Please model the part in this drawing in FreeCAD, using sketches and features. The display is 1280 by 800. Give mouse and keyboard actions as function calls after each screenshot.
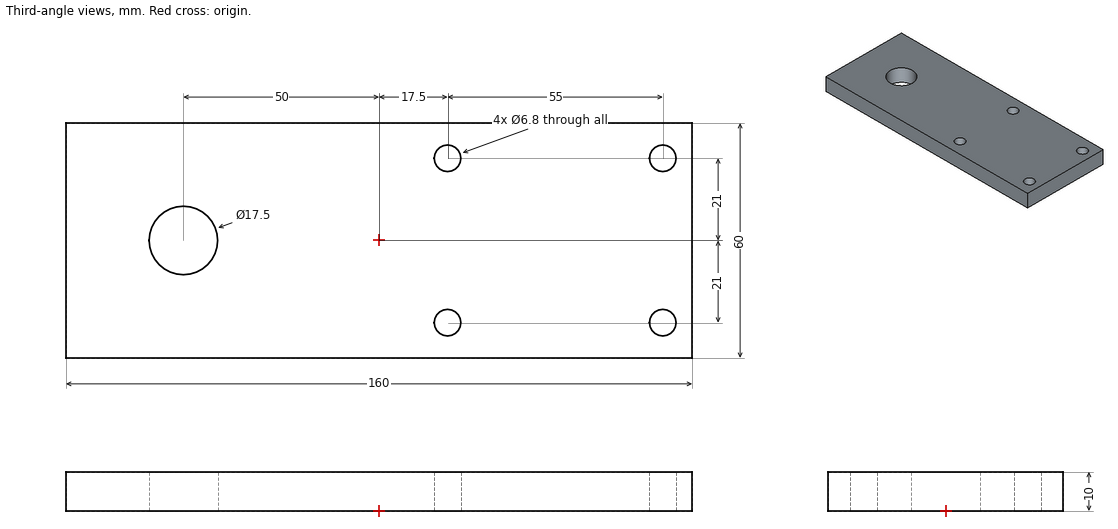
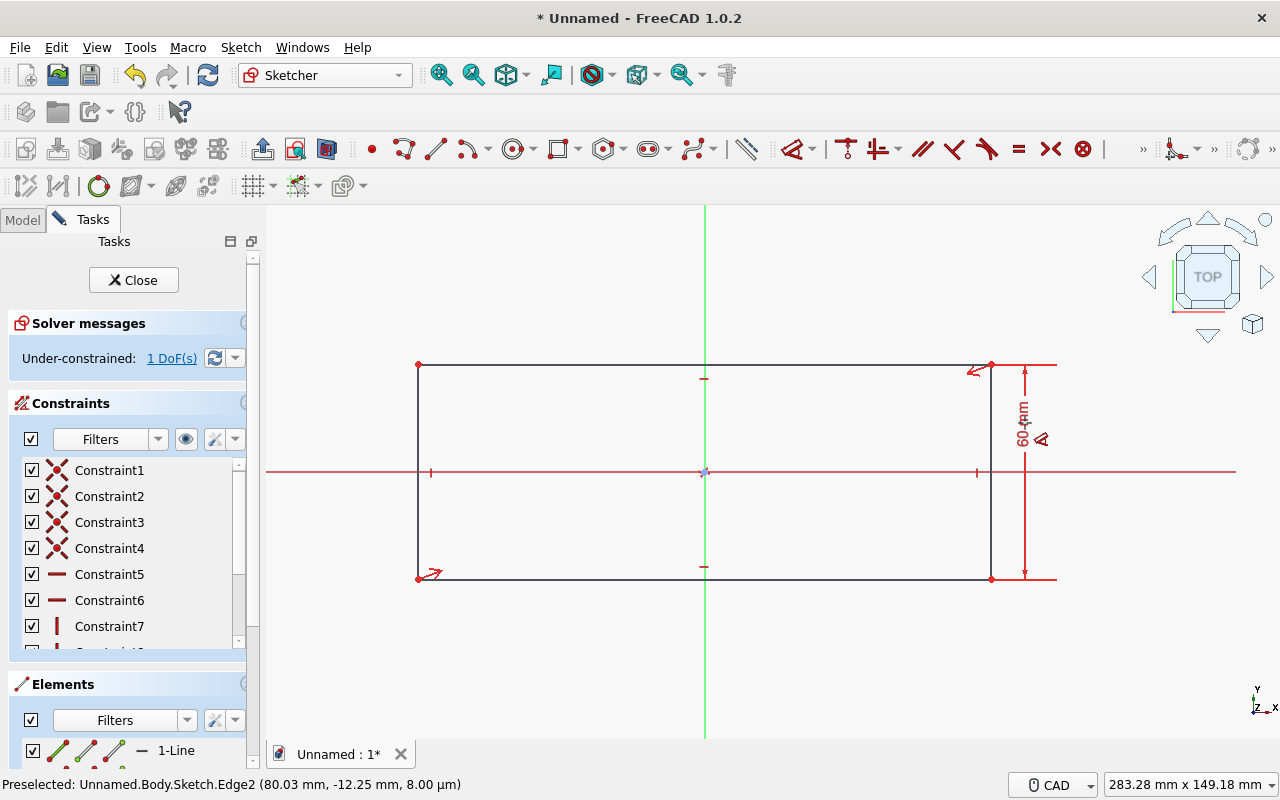
click(590, 580)
click(573, 614)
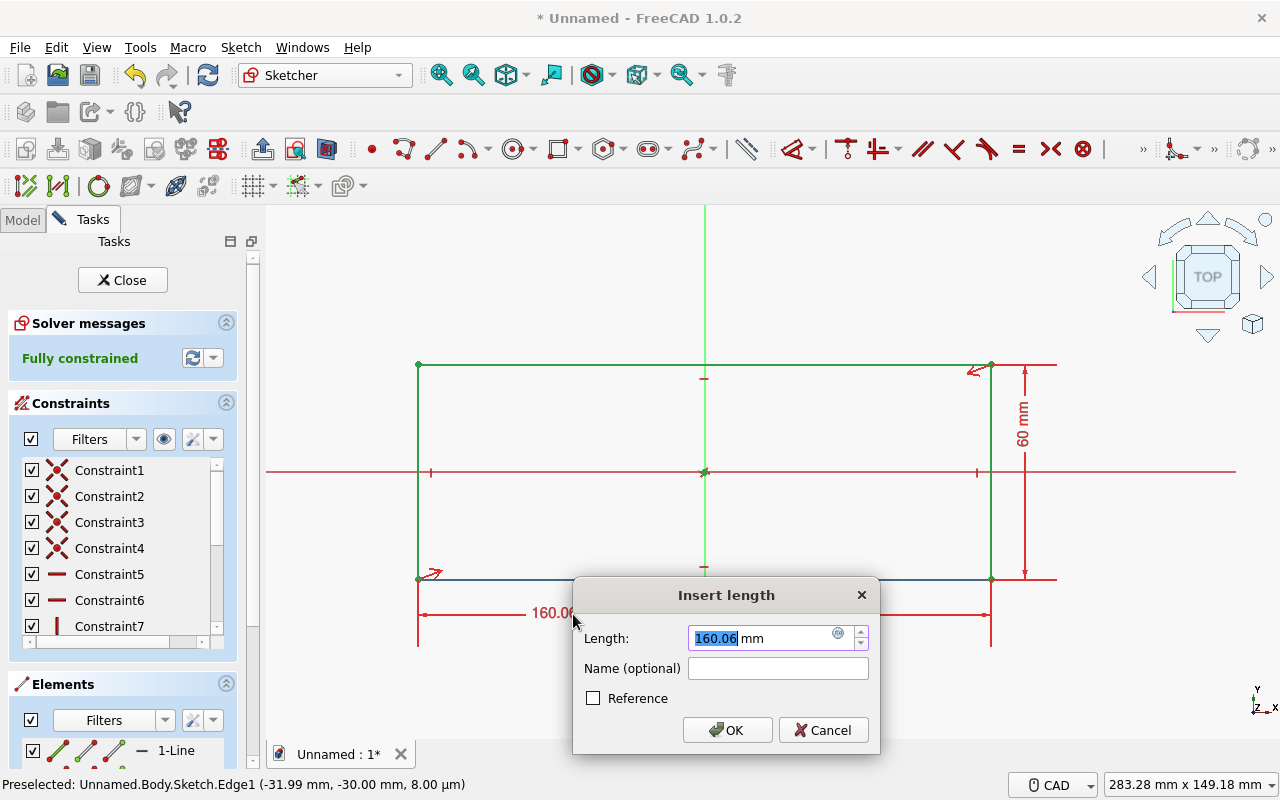
text(160)
key(Return)
key(Escape)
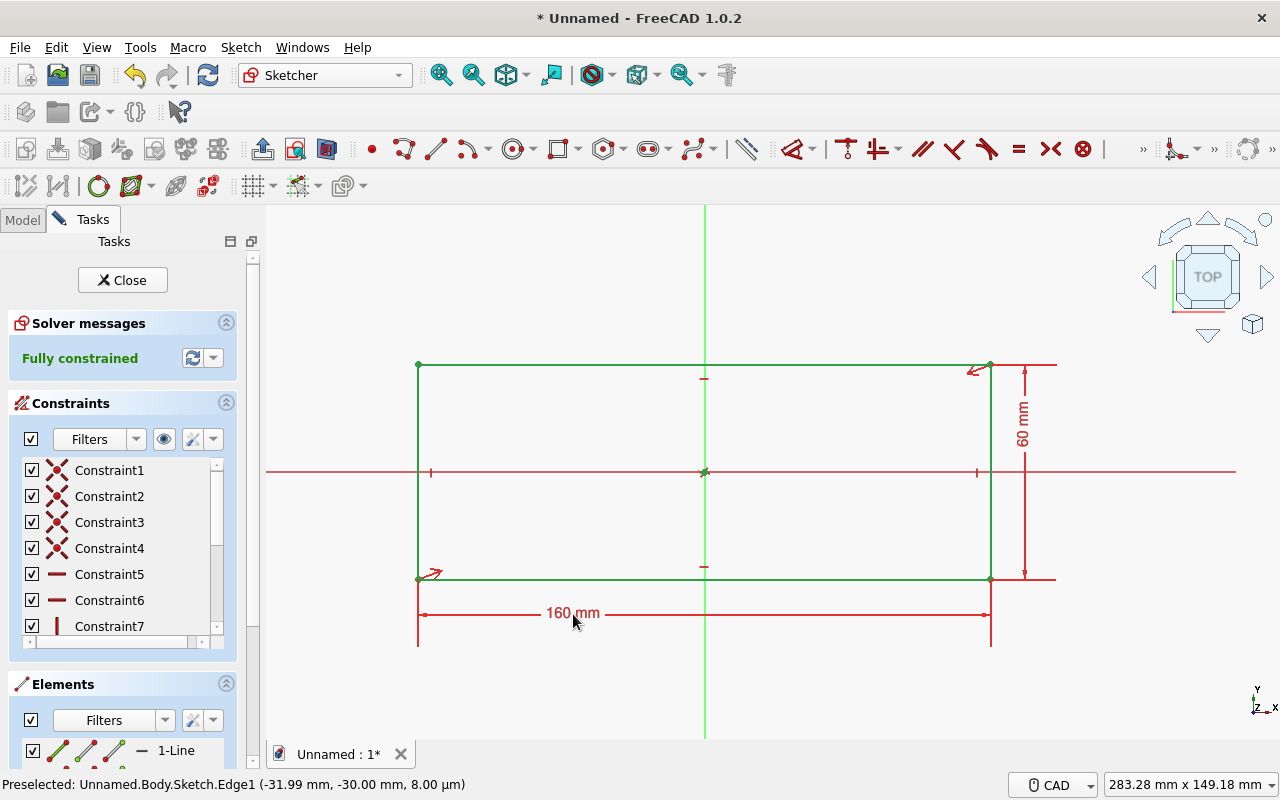
click(123, 280)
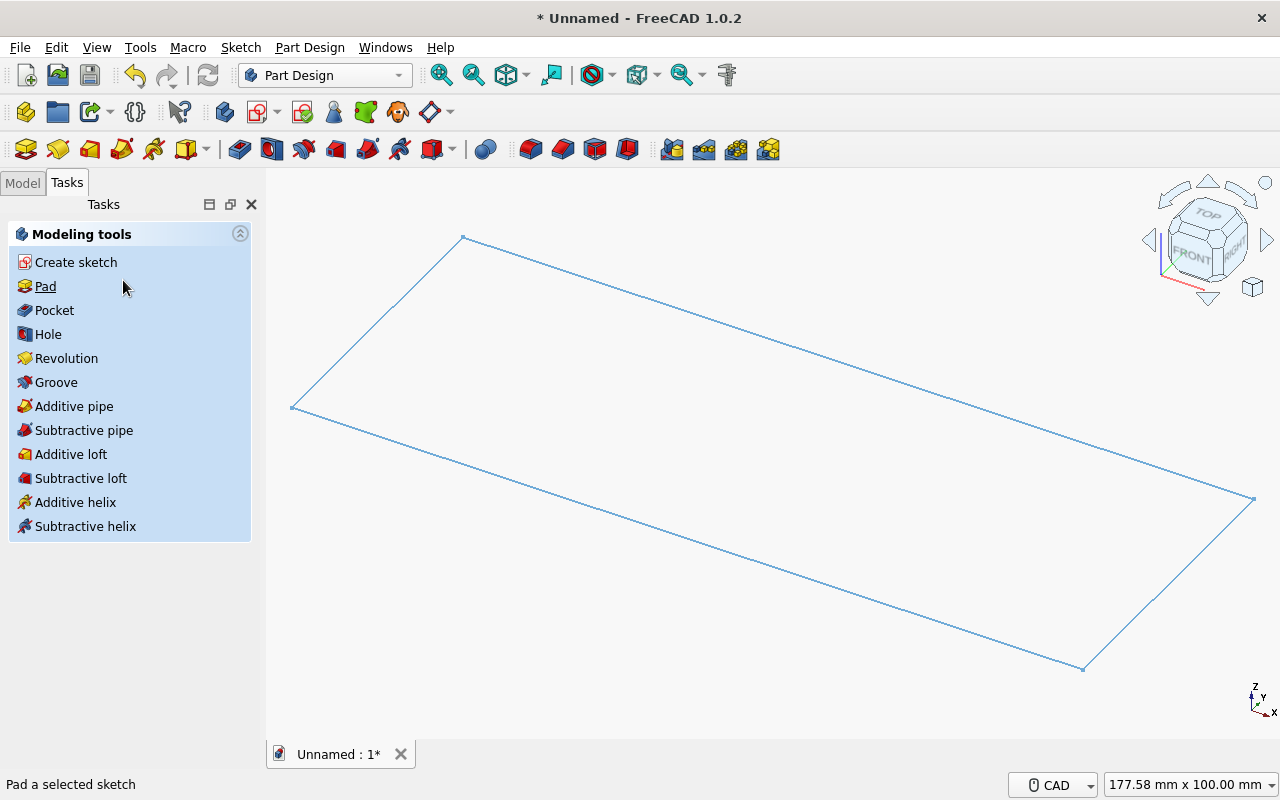
click(26, 150)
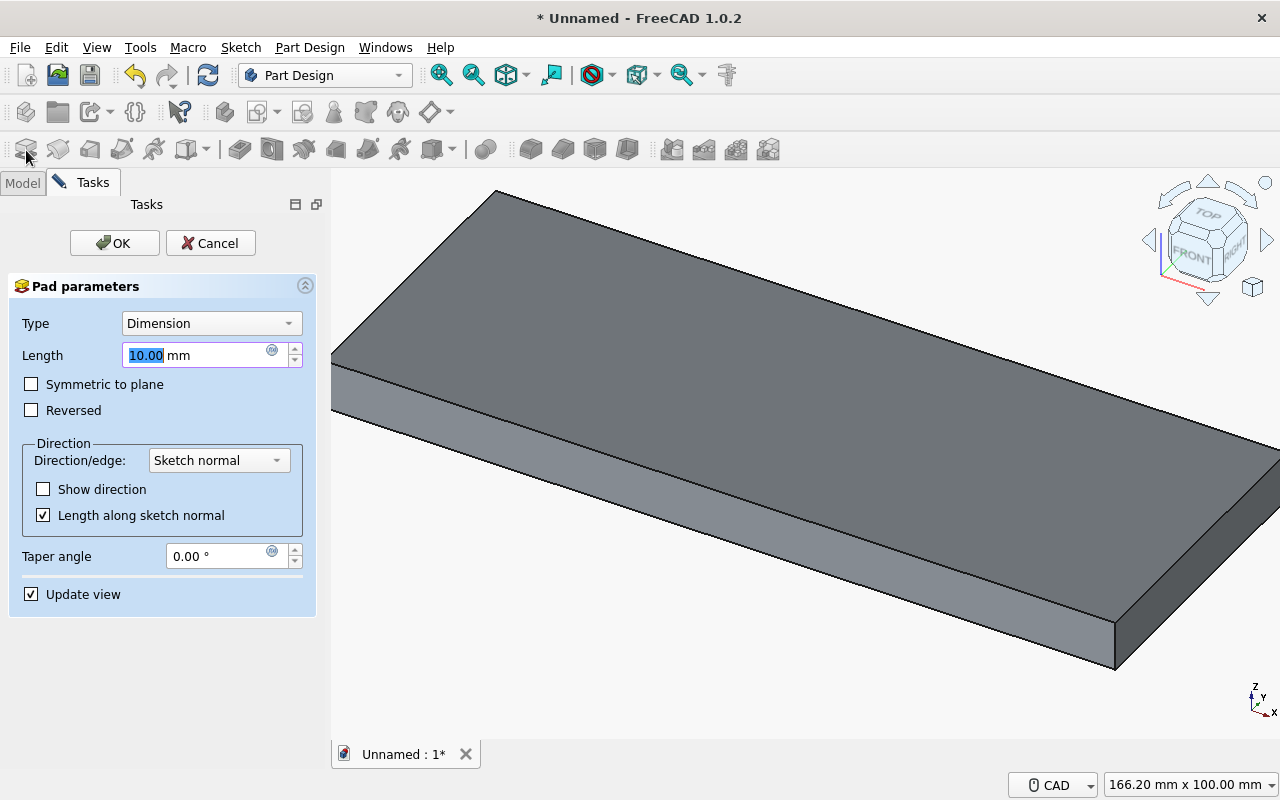
text(10)
key(Tab)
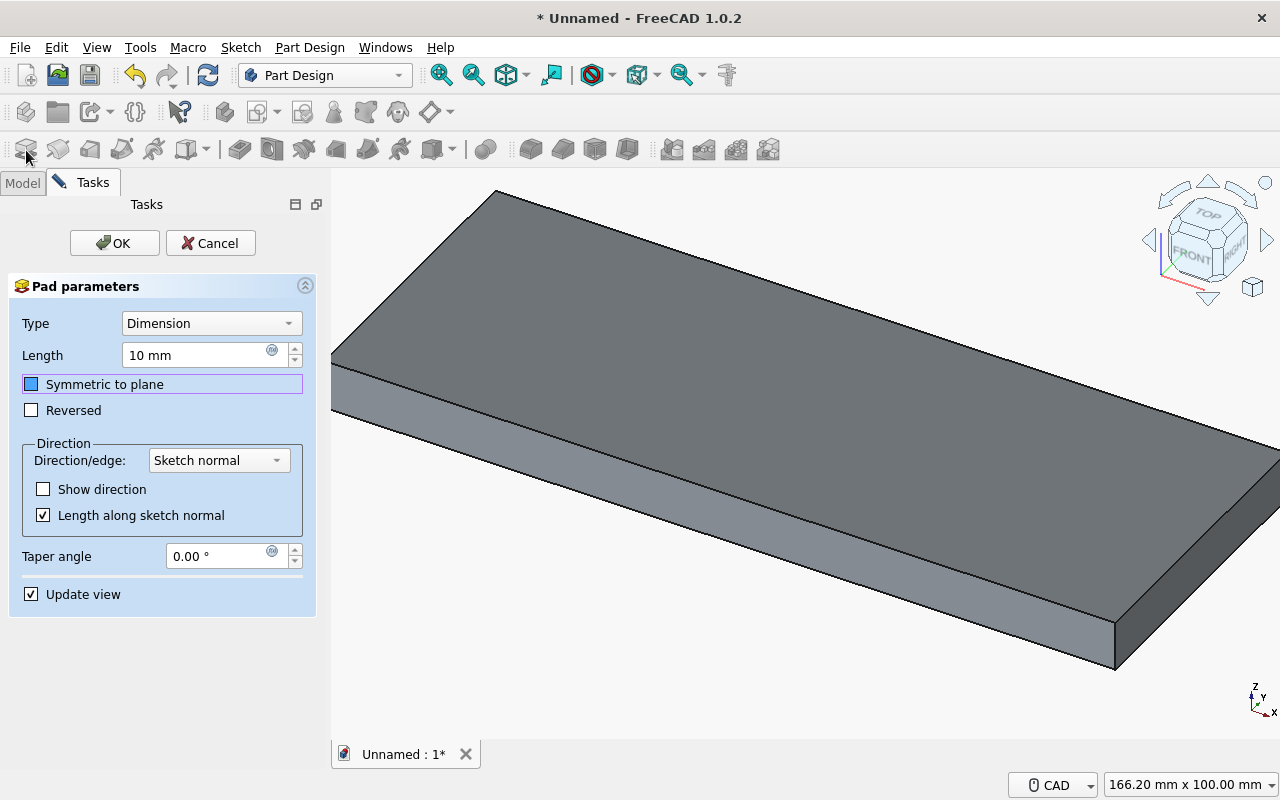
click(115, 243)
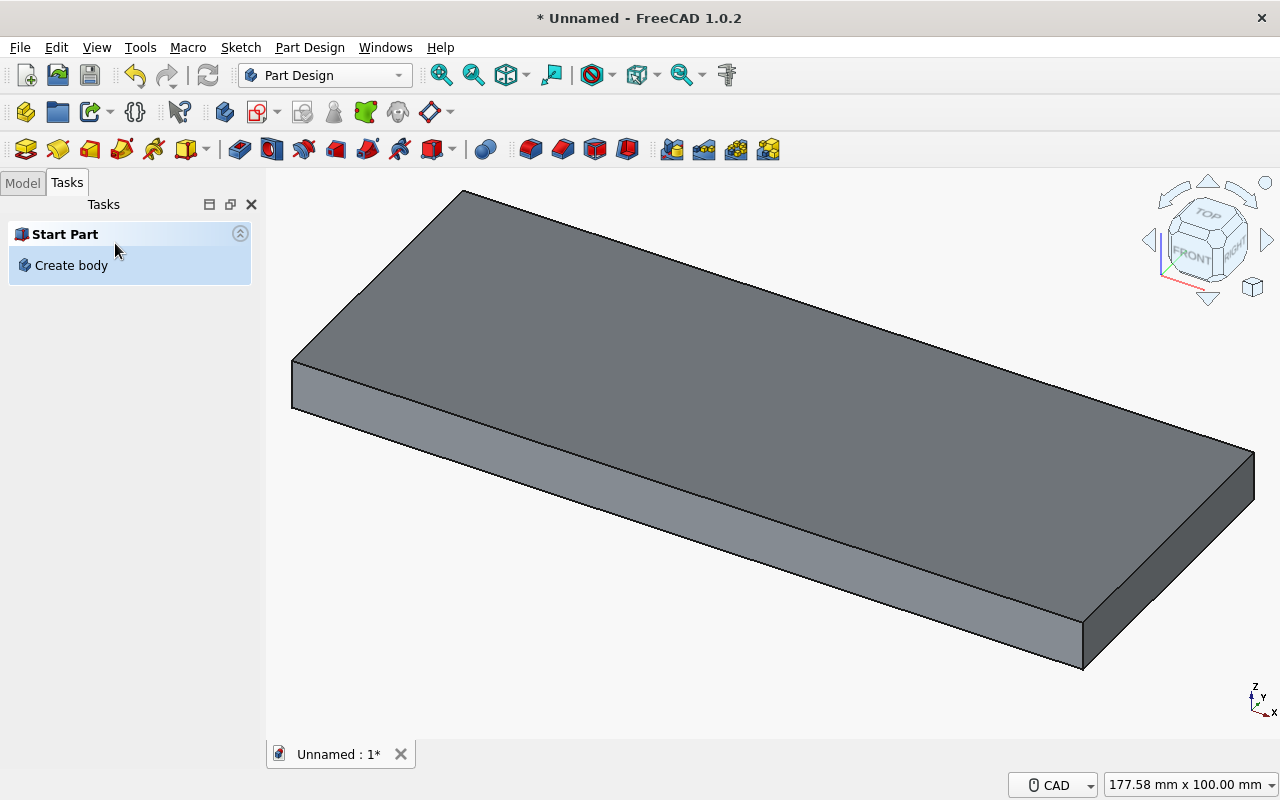
click(999, 481)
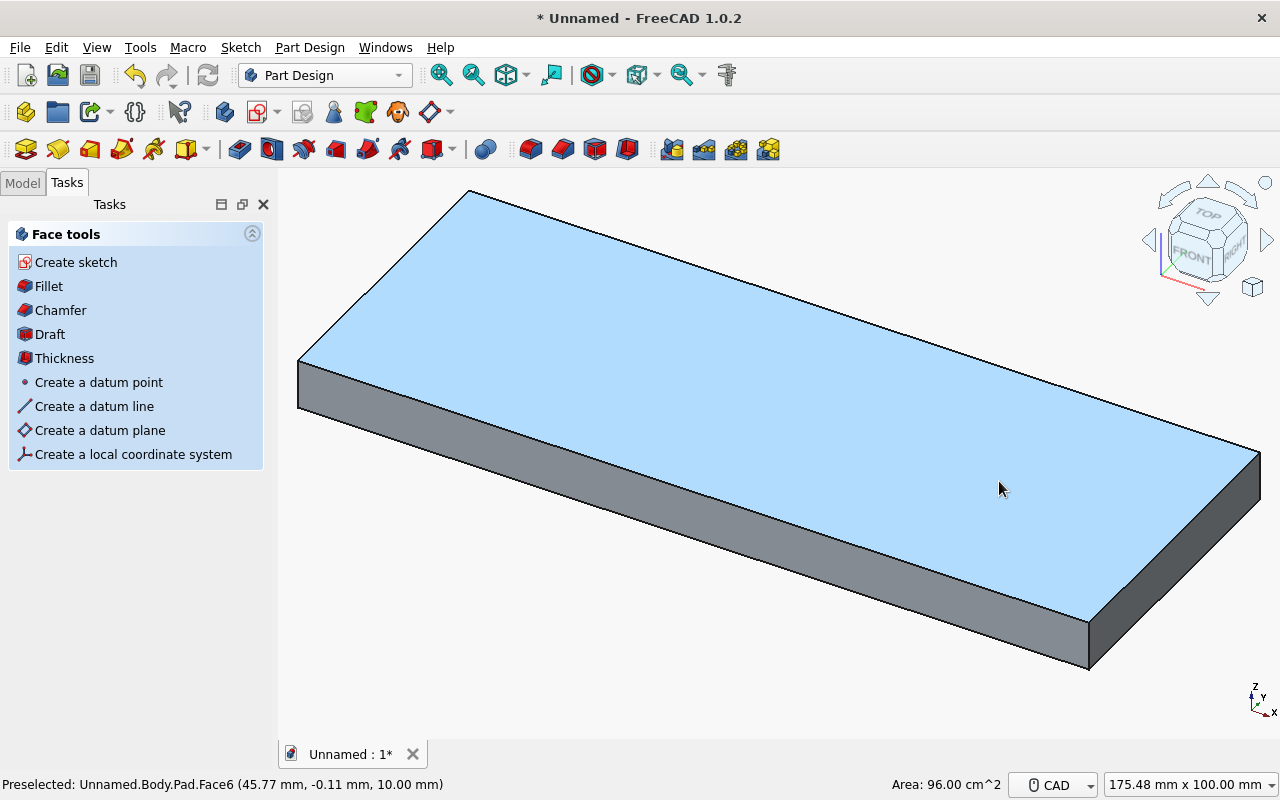
click(258, 112)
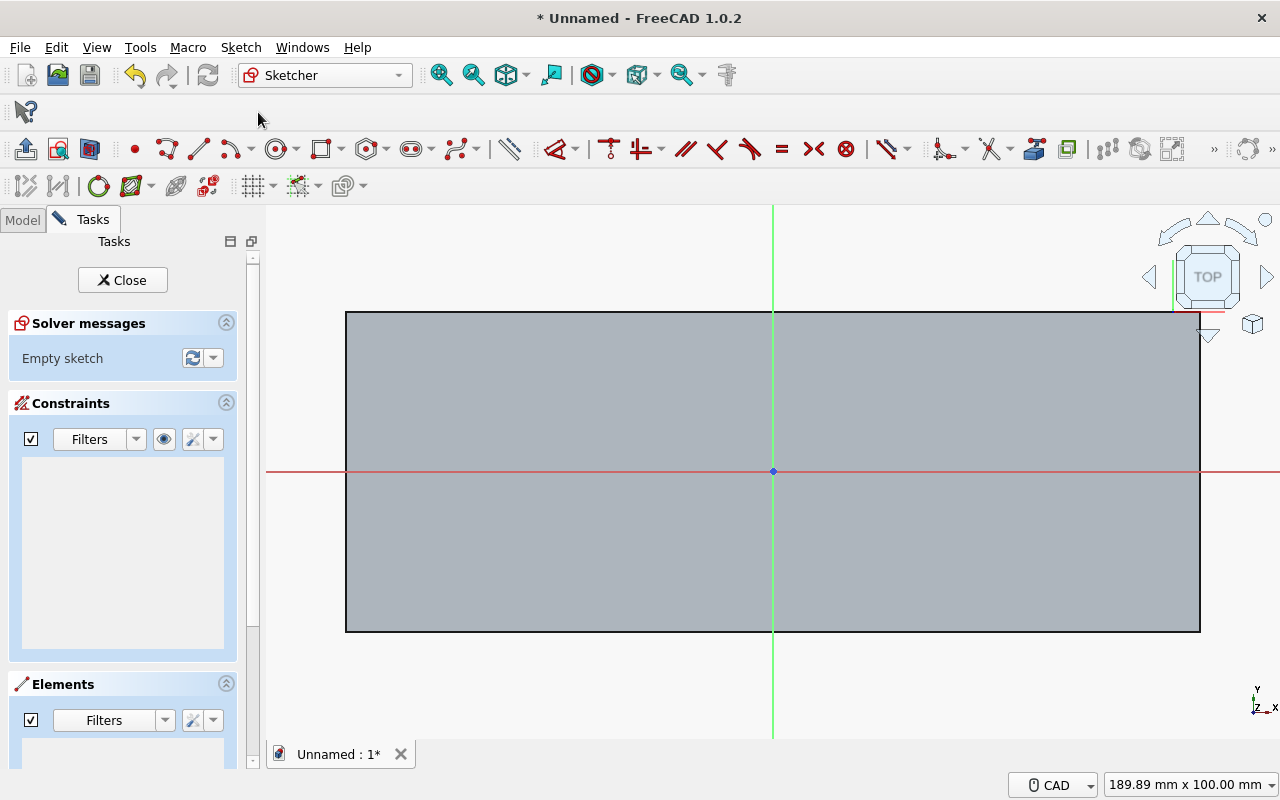
scroll(420, 472, up, 6)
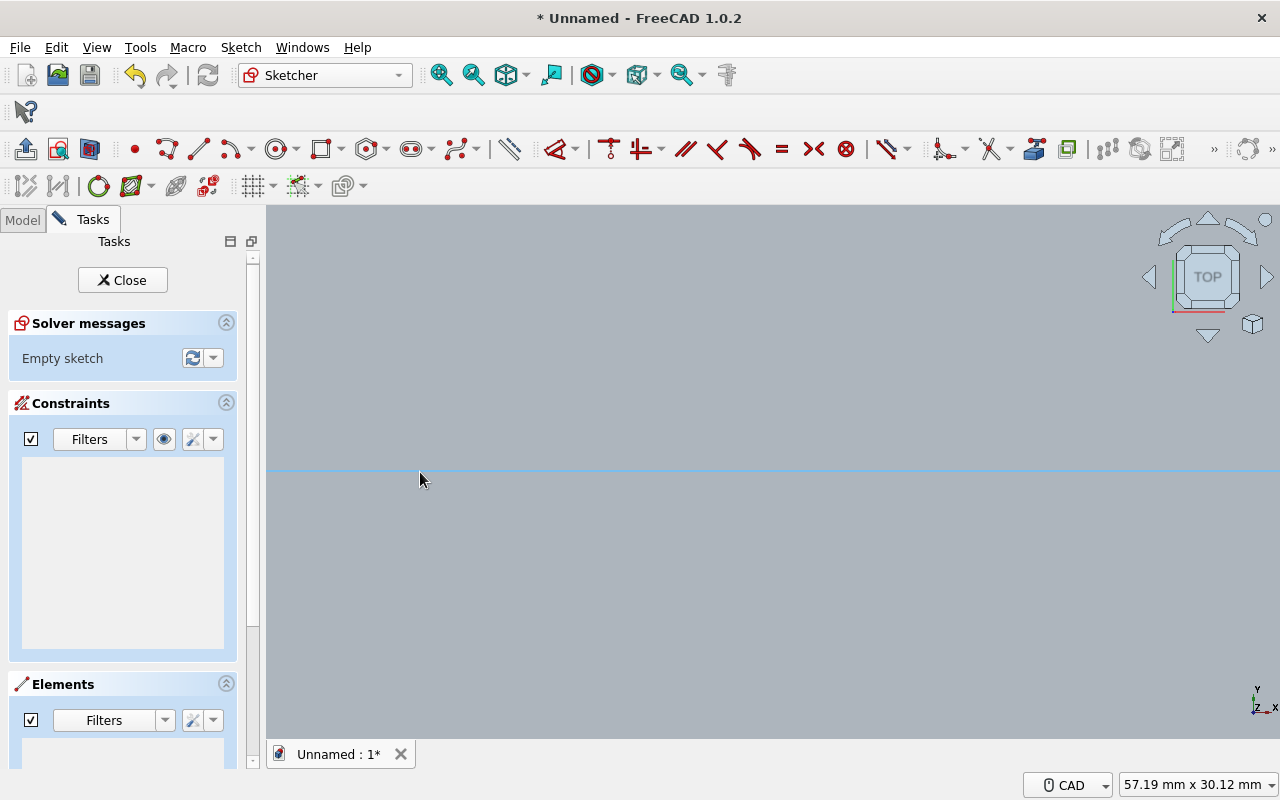
click(276, 150)